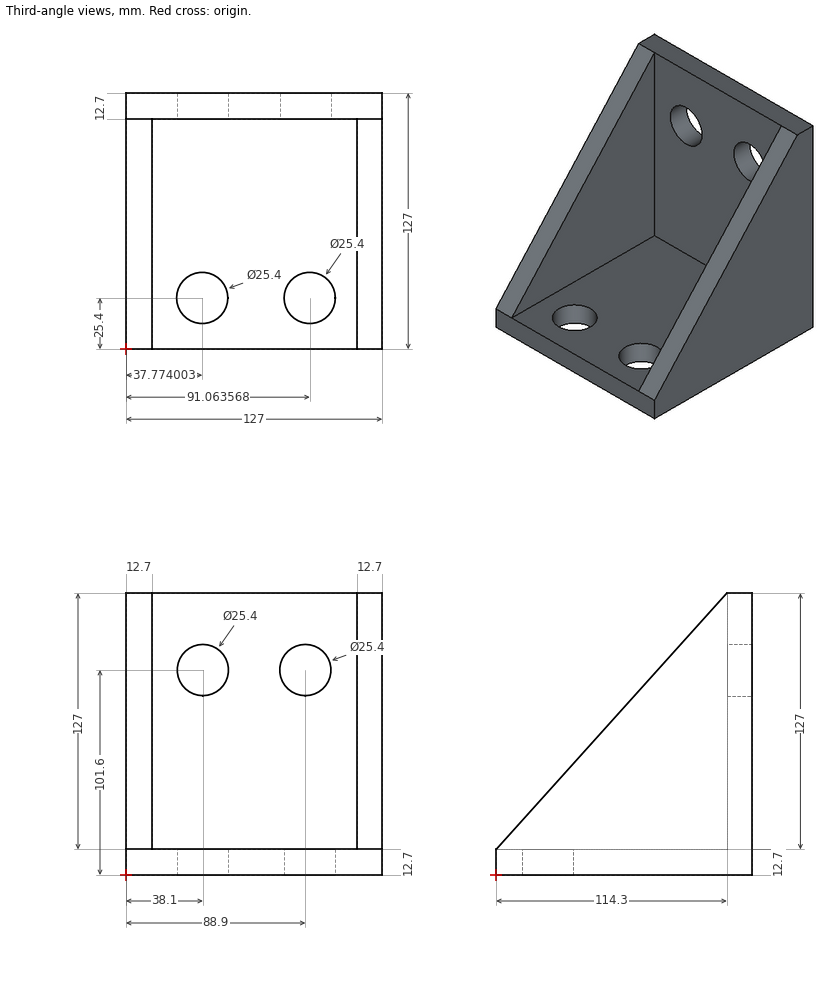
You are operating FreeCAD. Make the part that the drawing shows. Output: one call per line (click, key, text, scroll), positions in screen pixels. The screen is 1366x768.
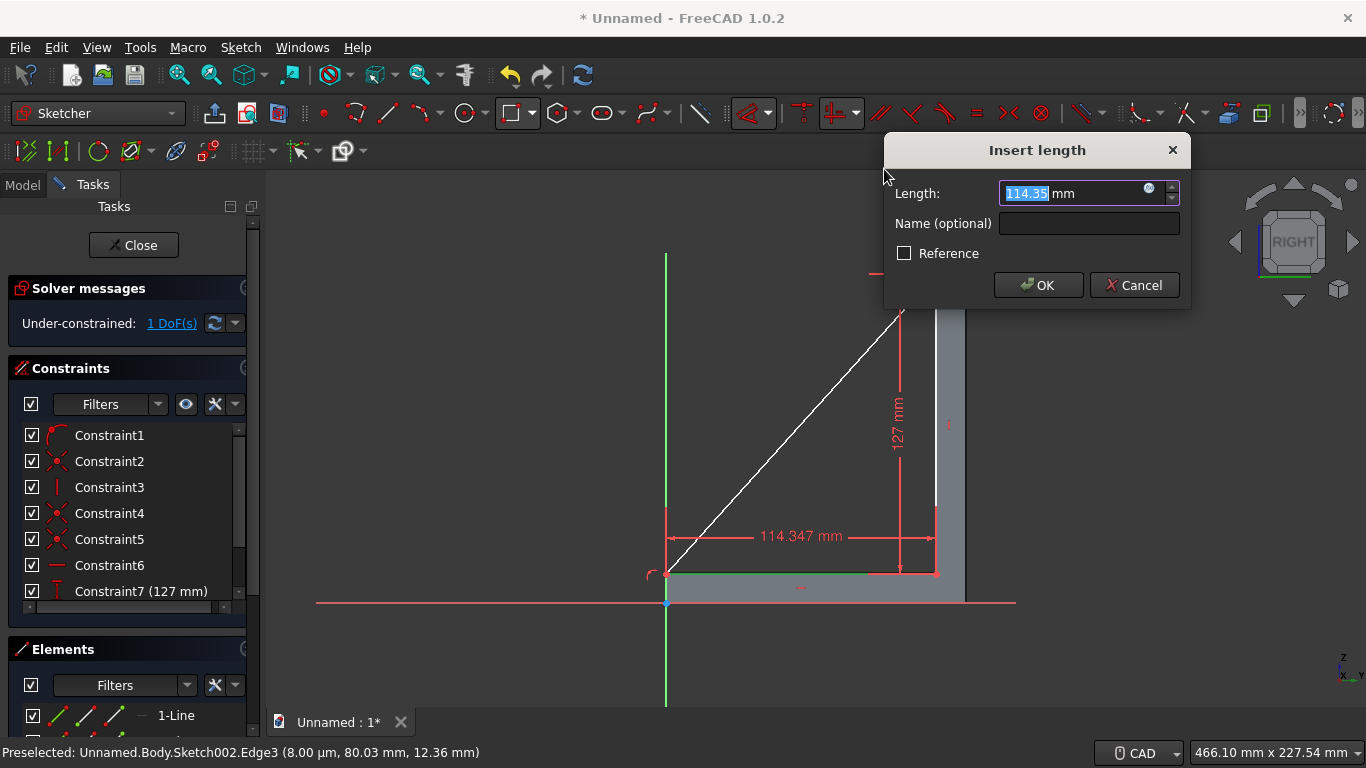
text(114.3)
key(Return)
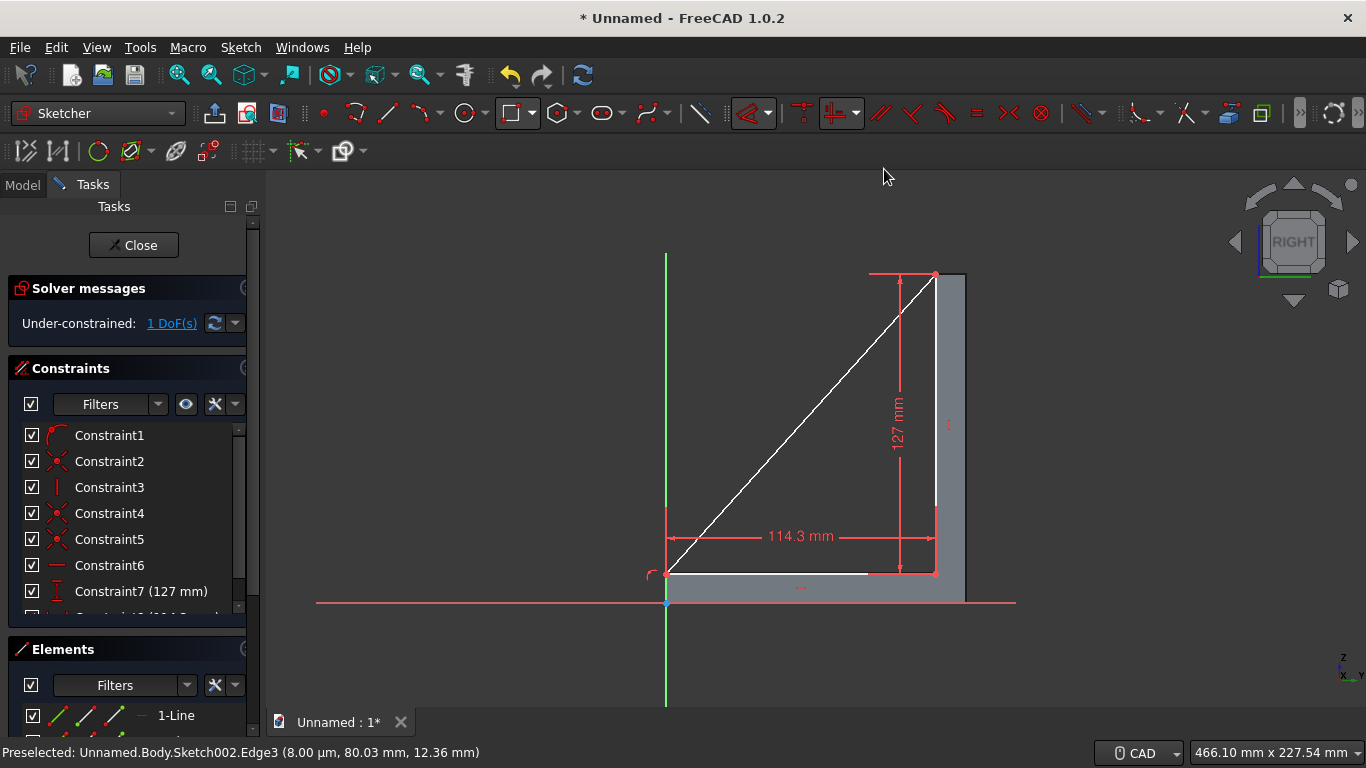
scroll(666, 574, up, 2)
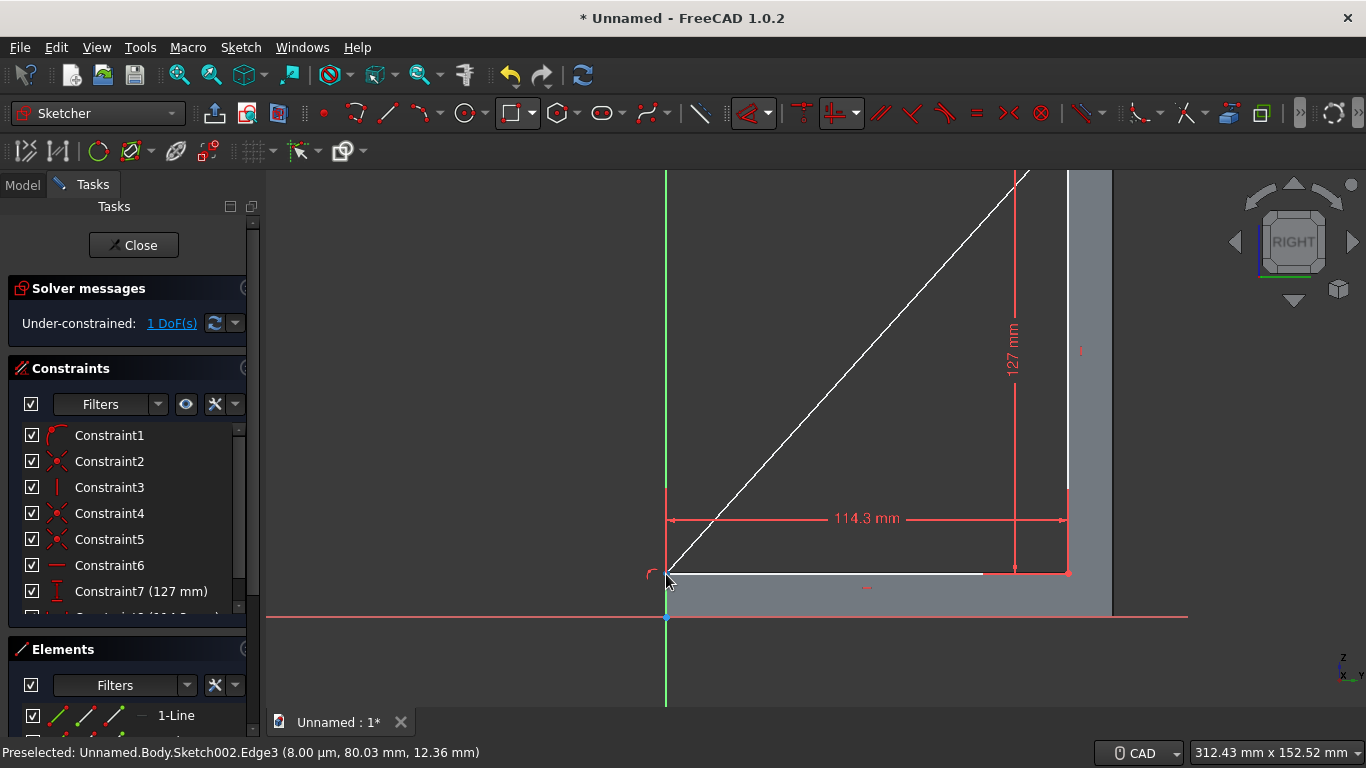
click(666, 574)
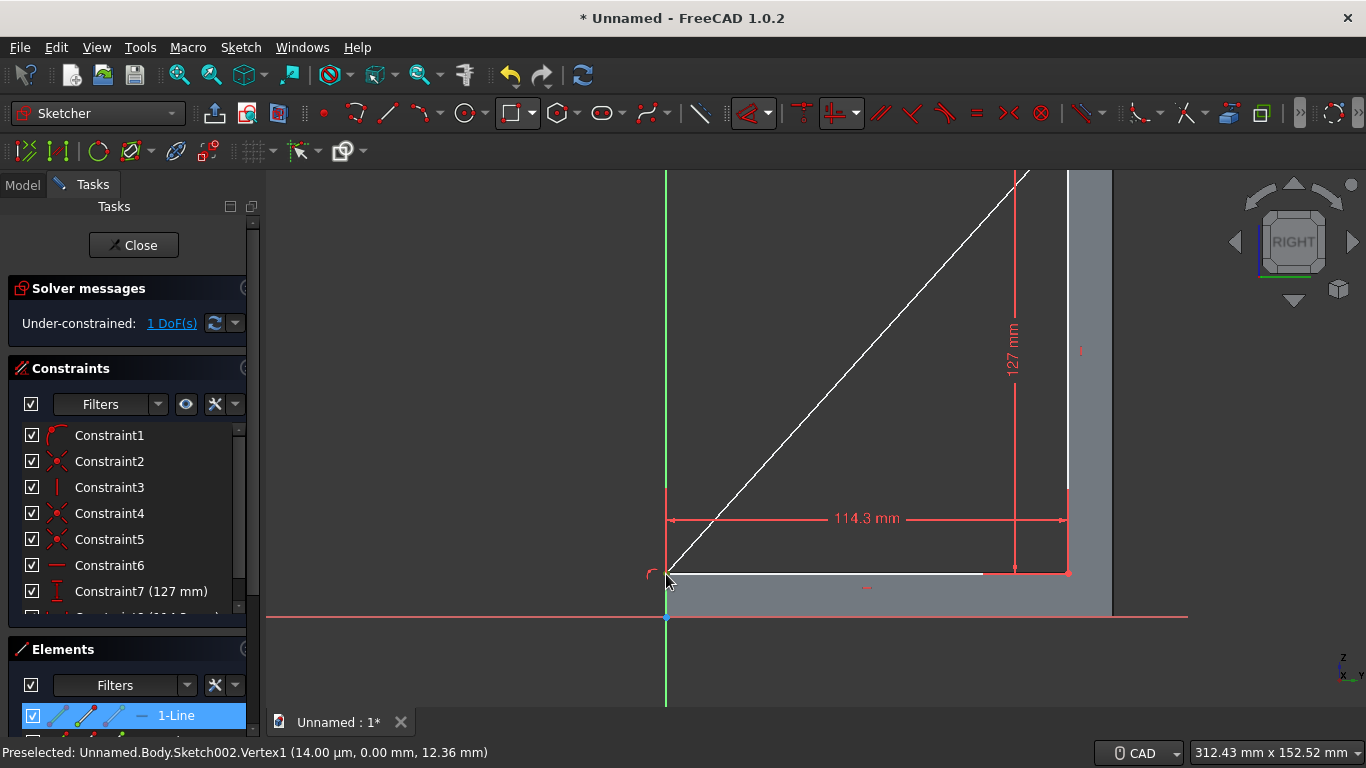
key(i)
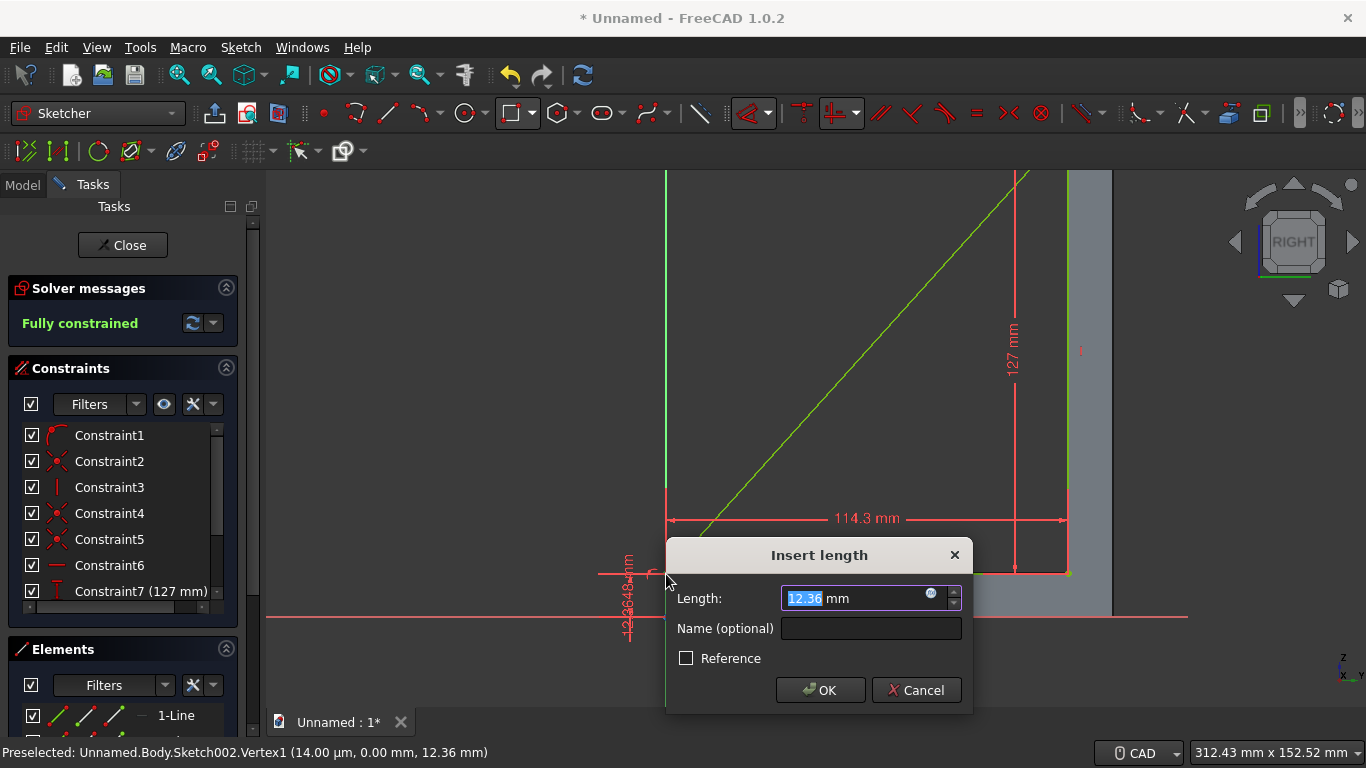
text(12.7)
key(Return)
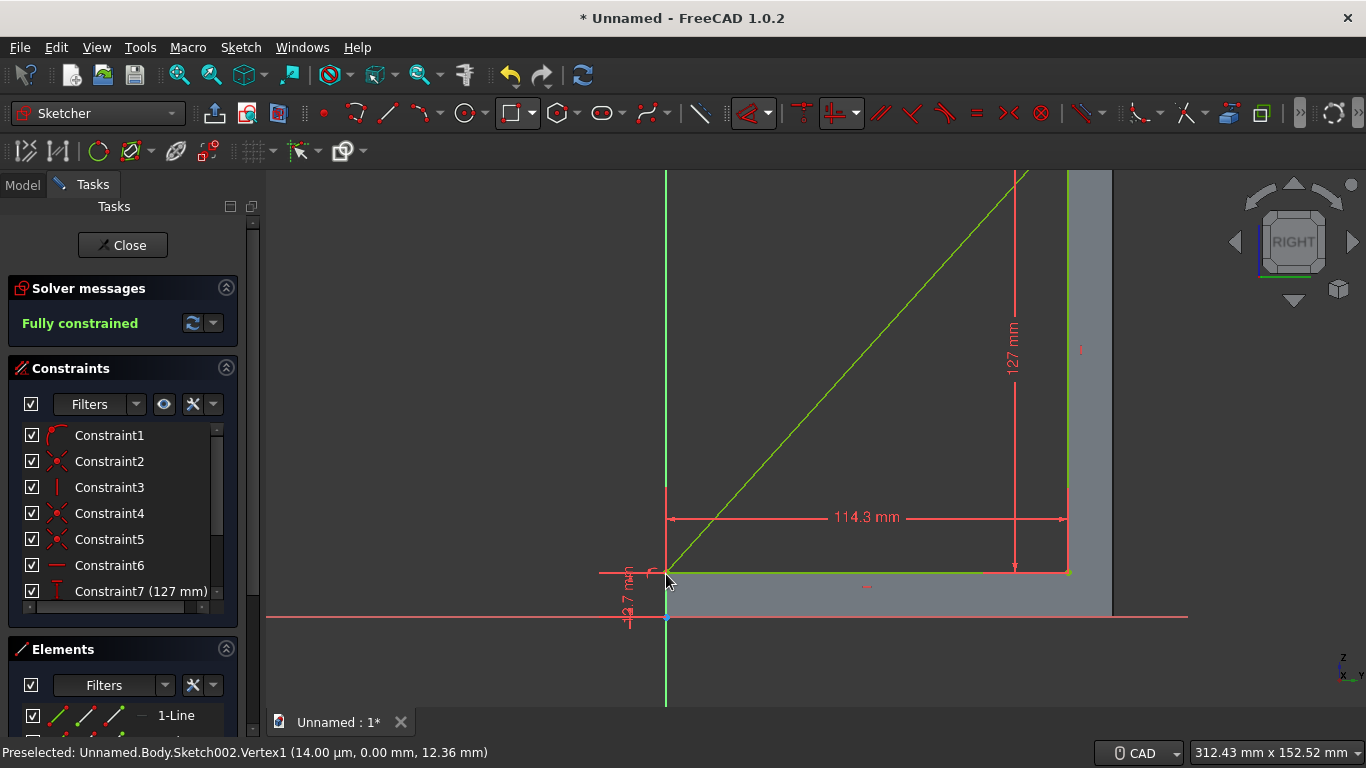
click(123, 245)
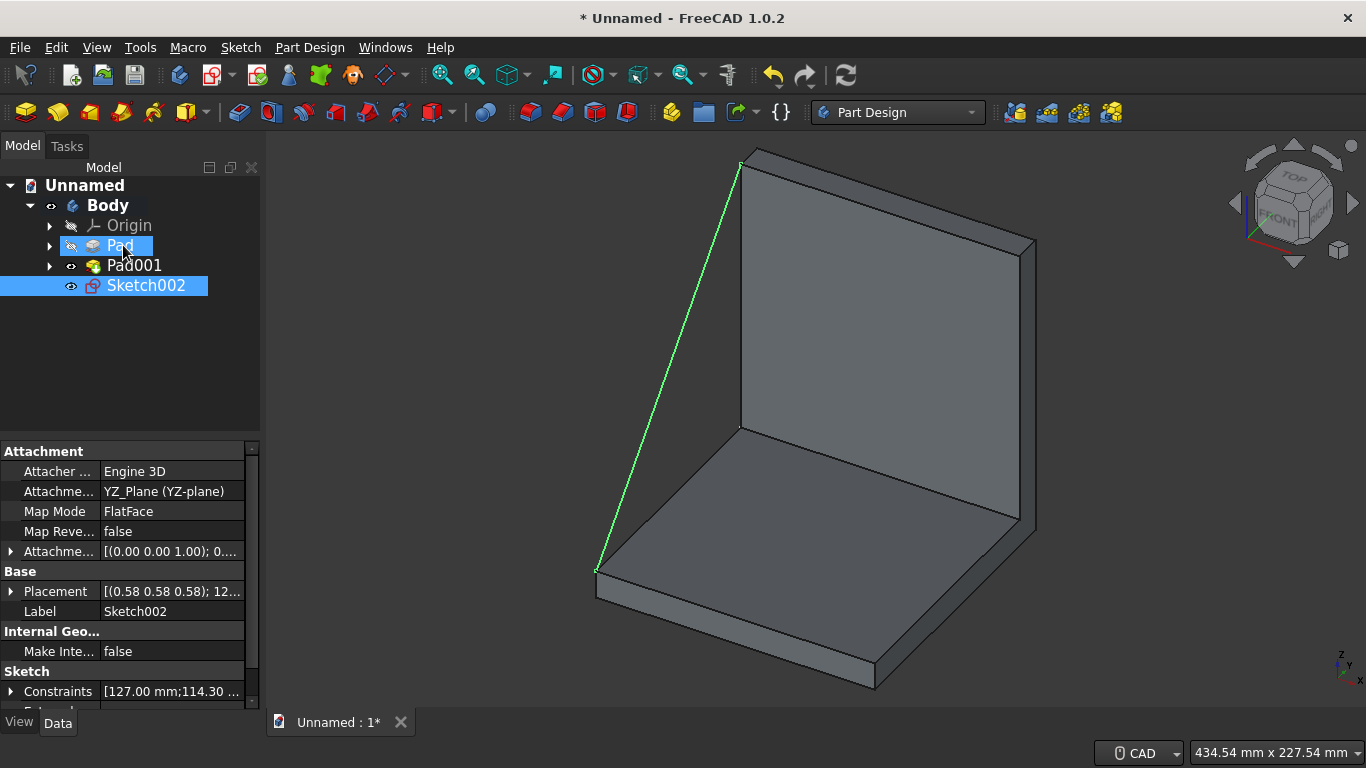
click(26, 112)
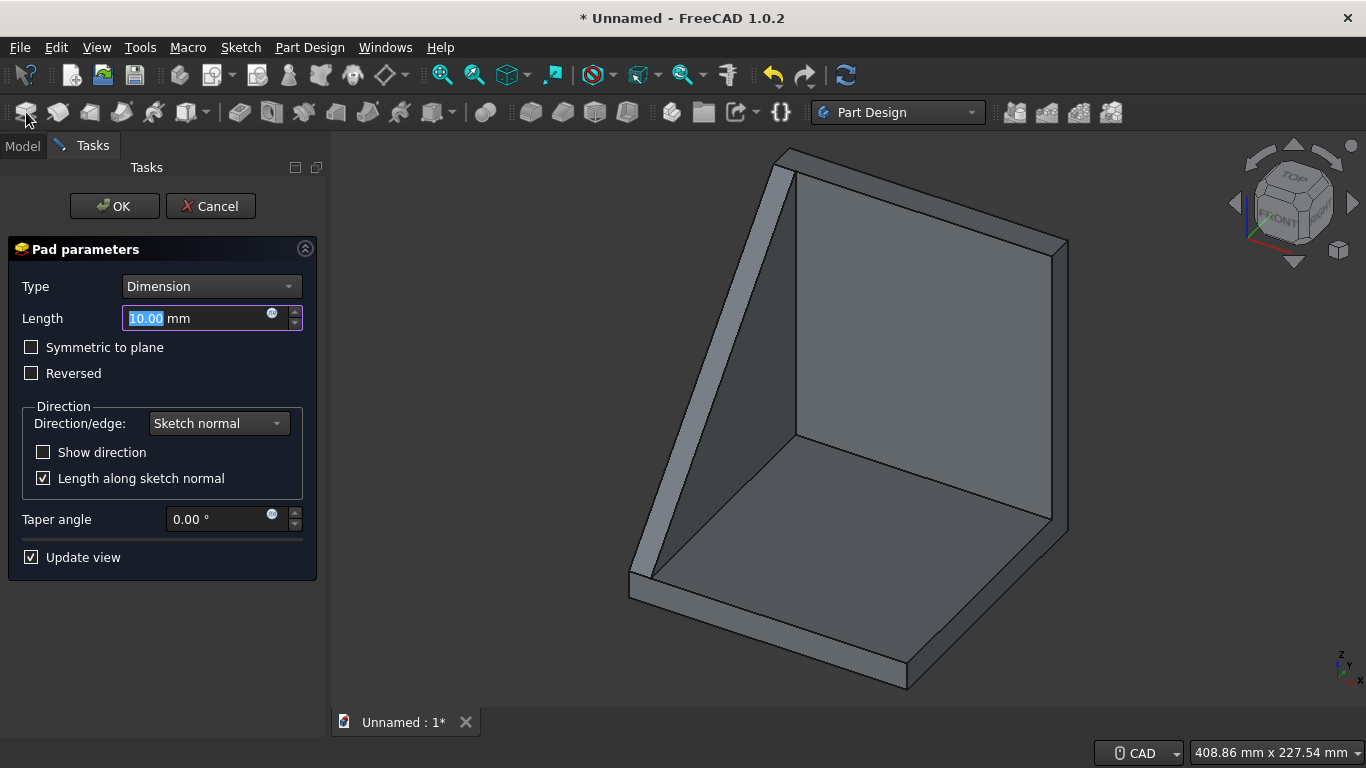
text(12.7)
key(Tab)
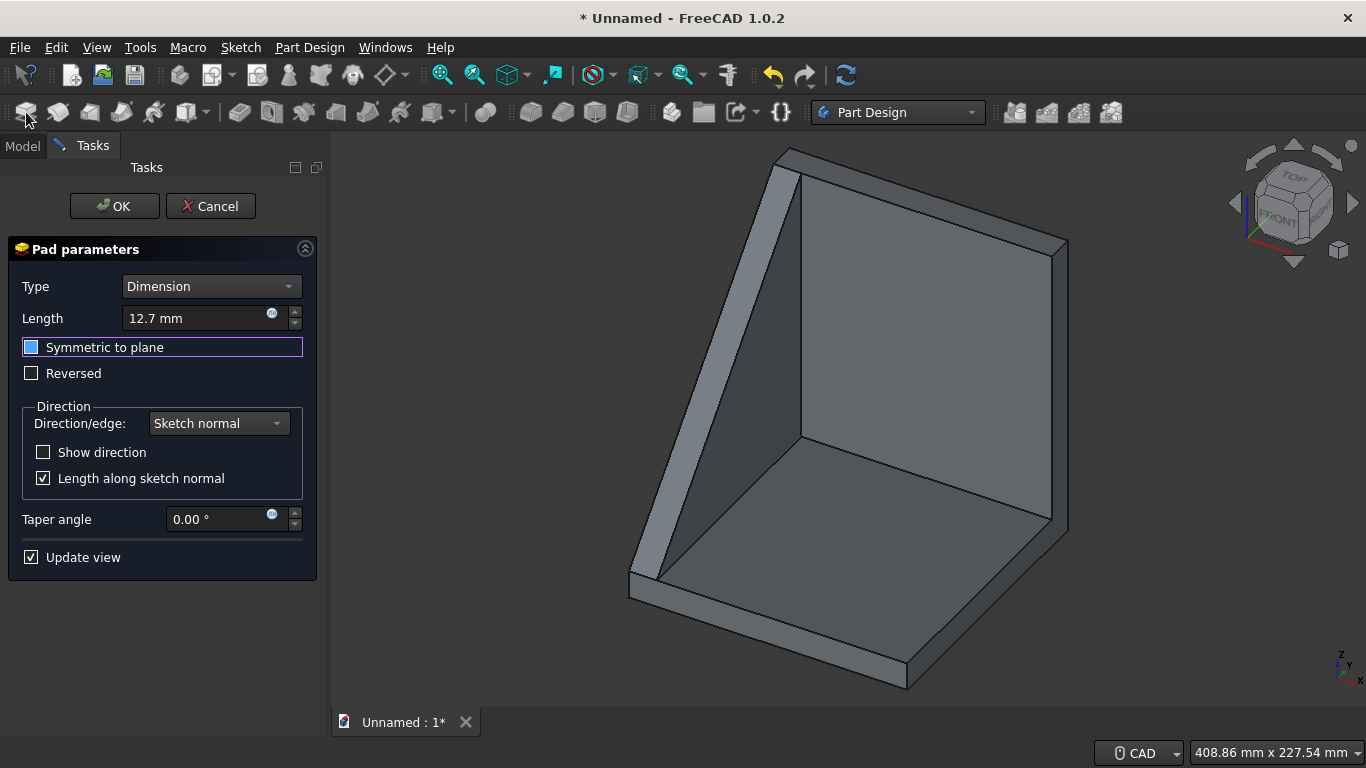
click(115, 206)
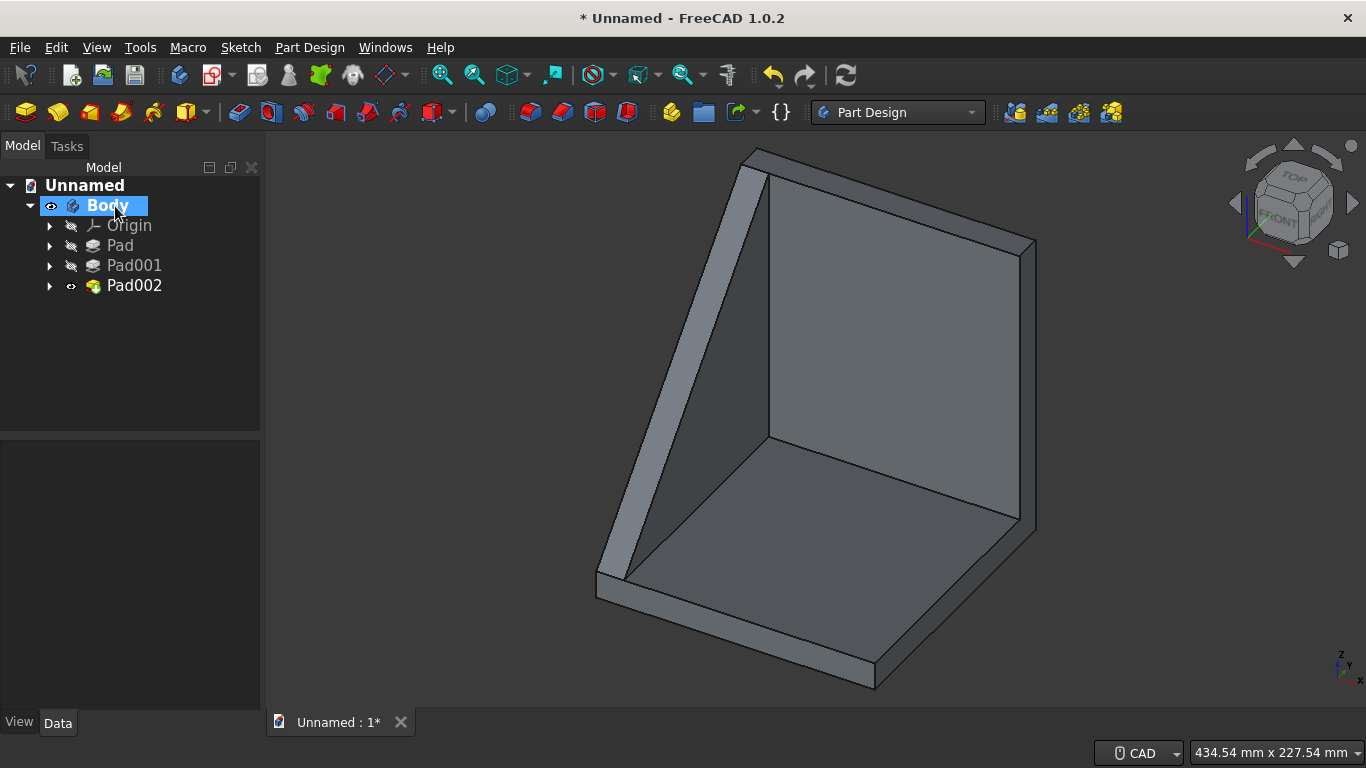
key(0)